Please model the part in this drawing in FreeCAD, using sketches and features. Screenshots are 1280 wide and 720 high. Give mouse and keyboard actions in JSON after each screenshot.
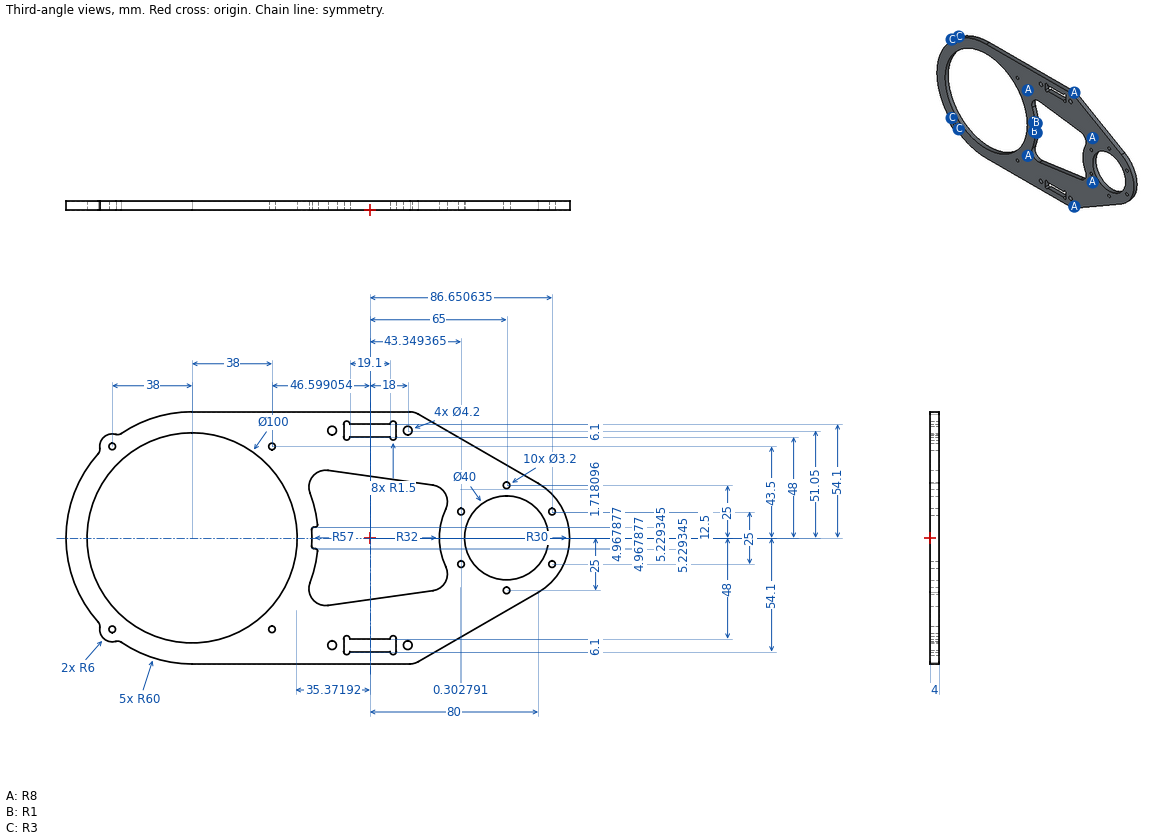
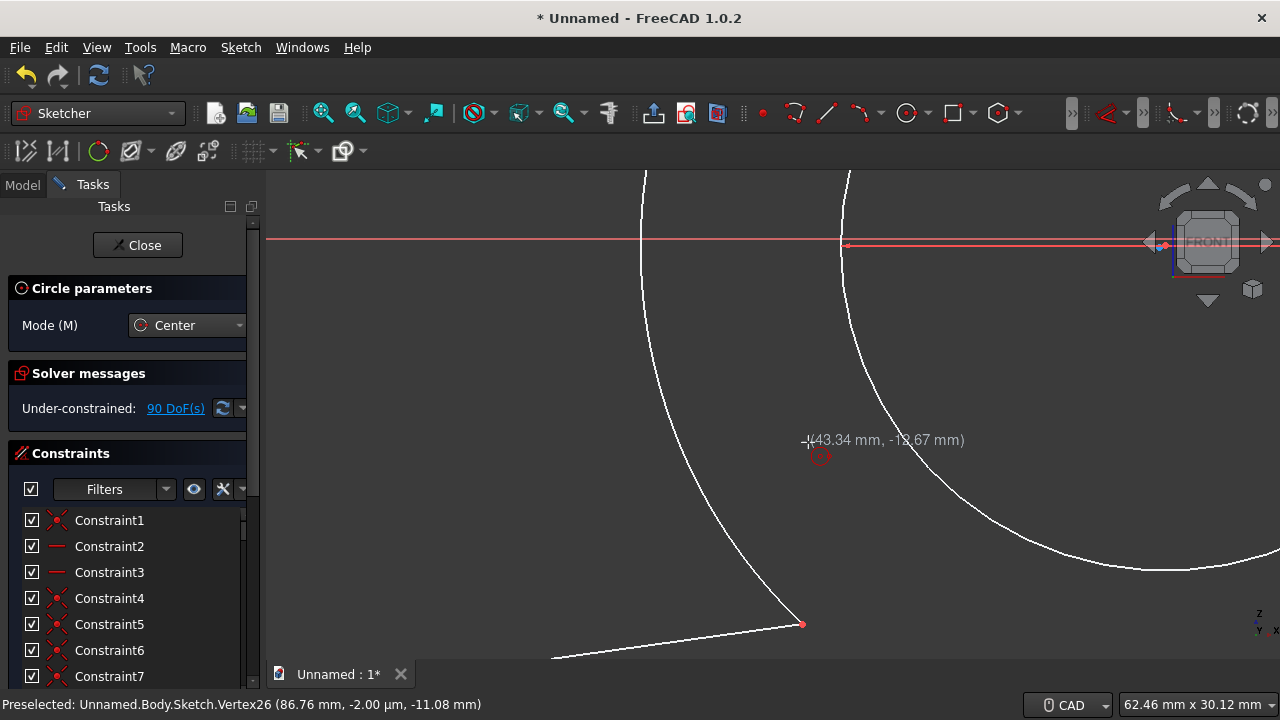
{"action": "scroll", "coordinate": [862, 442], "scroll_direction": "down", "scroll_amount": 10}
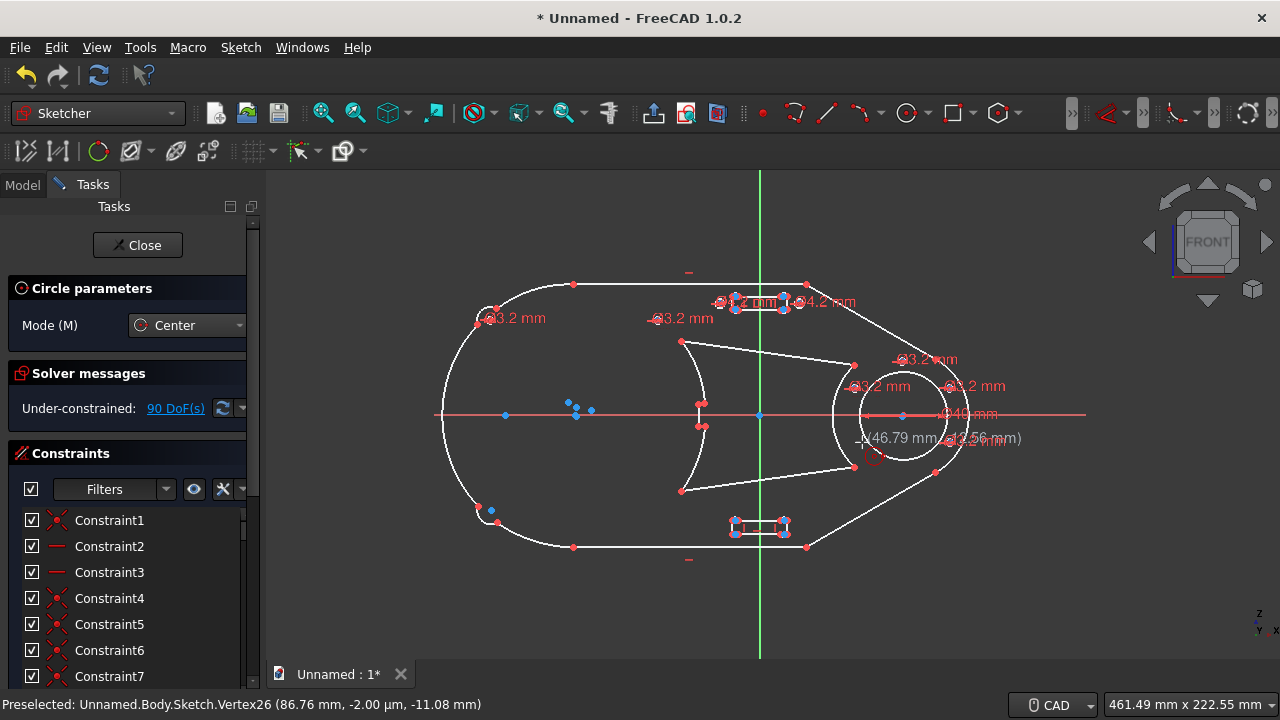
{"action": "scroll", "coordinate": [855, 442], "scroll_direction": "up", "scroll_amount": 2}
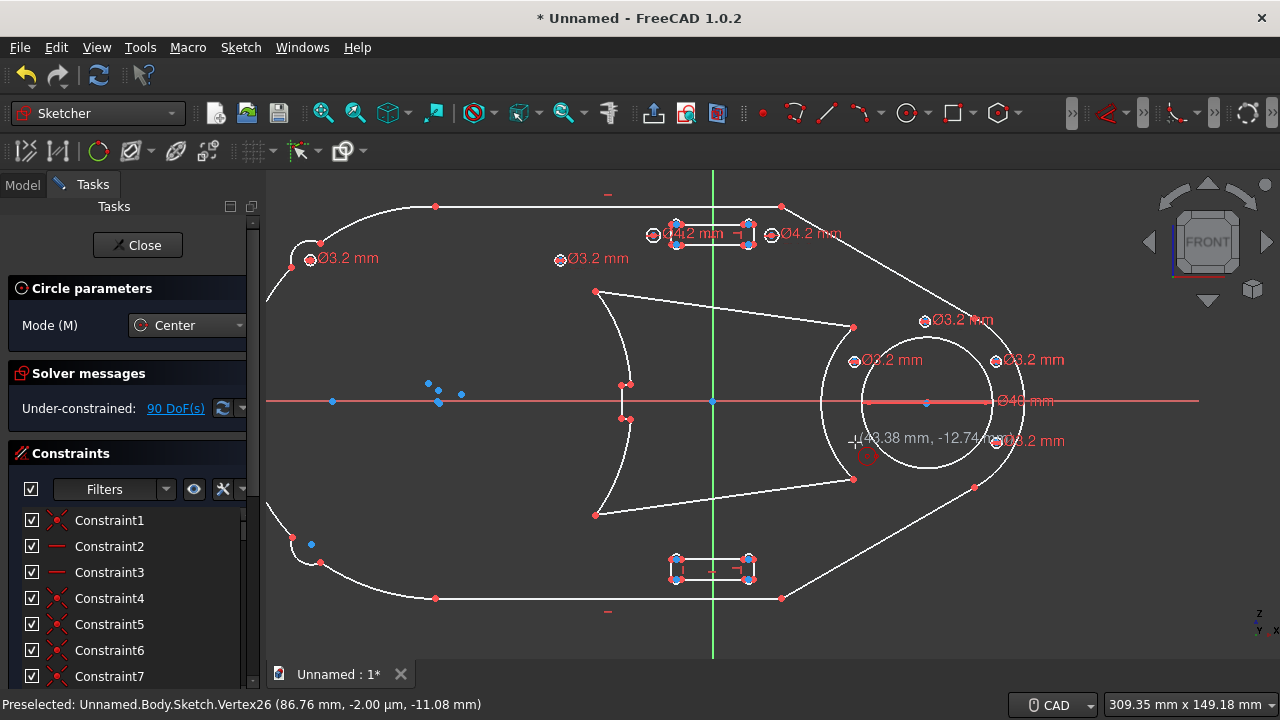
{"action": "left_click", "coordinate": [855, 442]}
{"action": "mouse_move", "coordinate": [851, 439]}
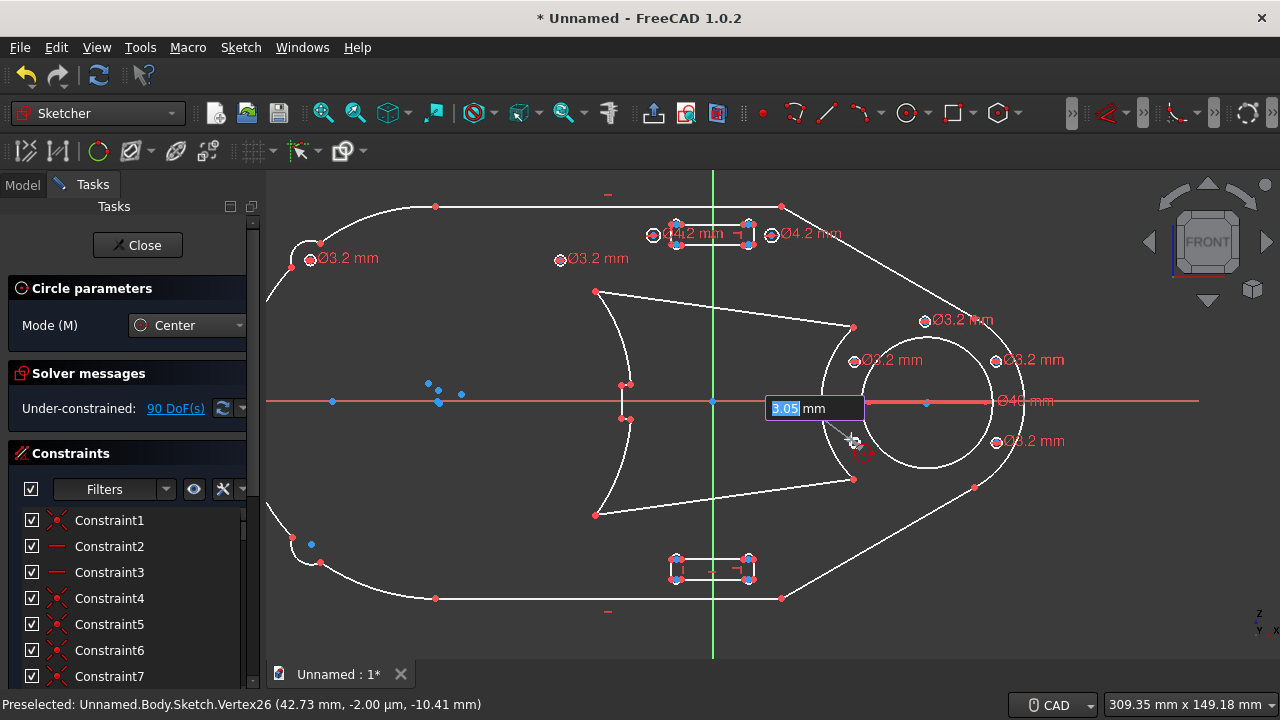
{"action": "type", "text": "3.2"}
{"action": "key", "text": "Return"}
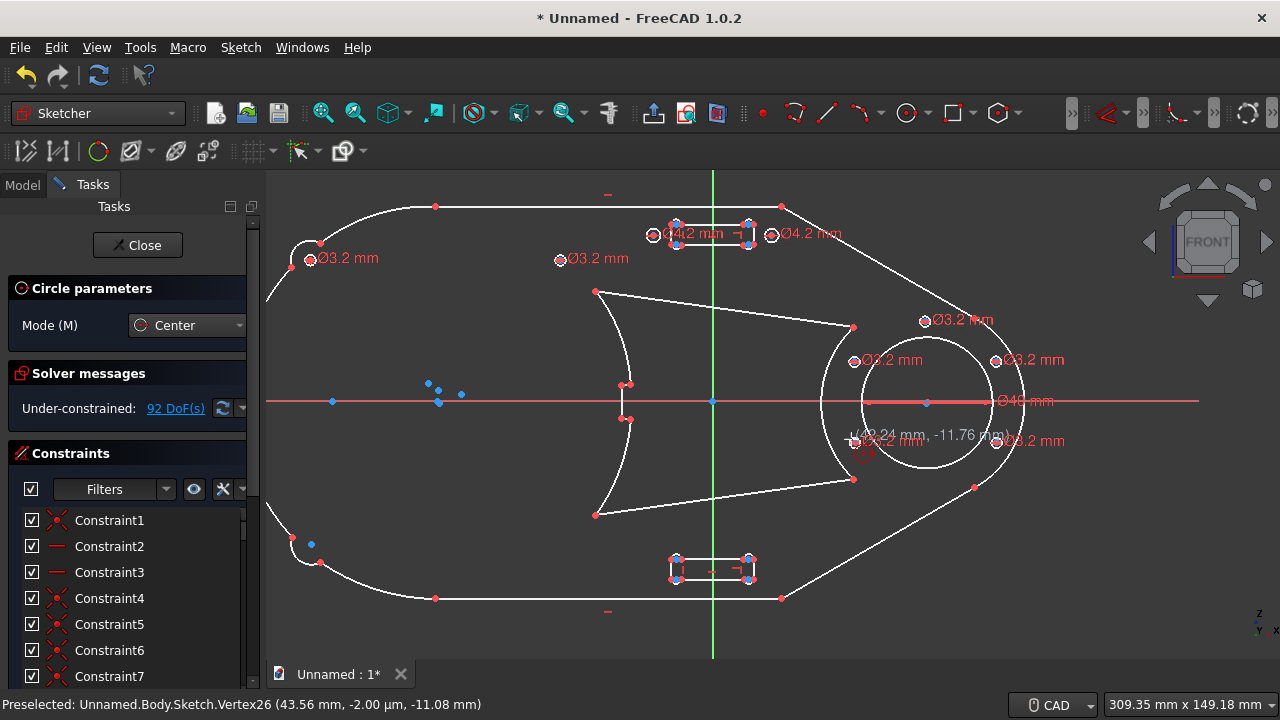
{"action": "scroll", "coordinate": [926, 483], "scroll_direction": "up", "scroll_amount": 8}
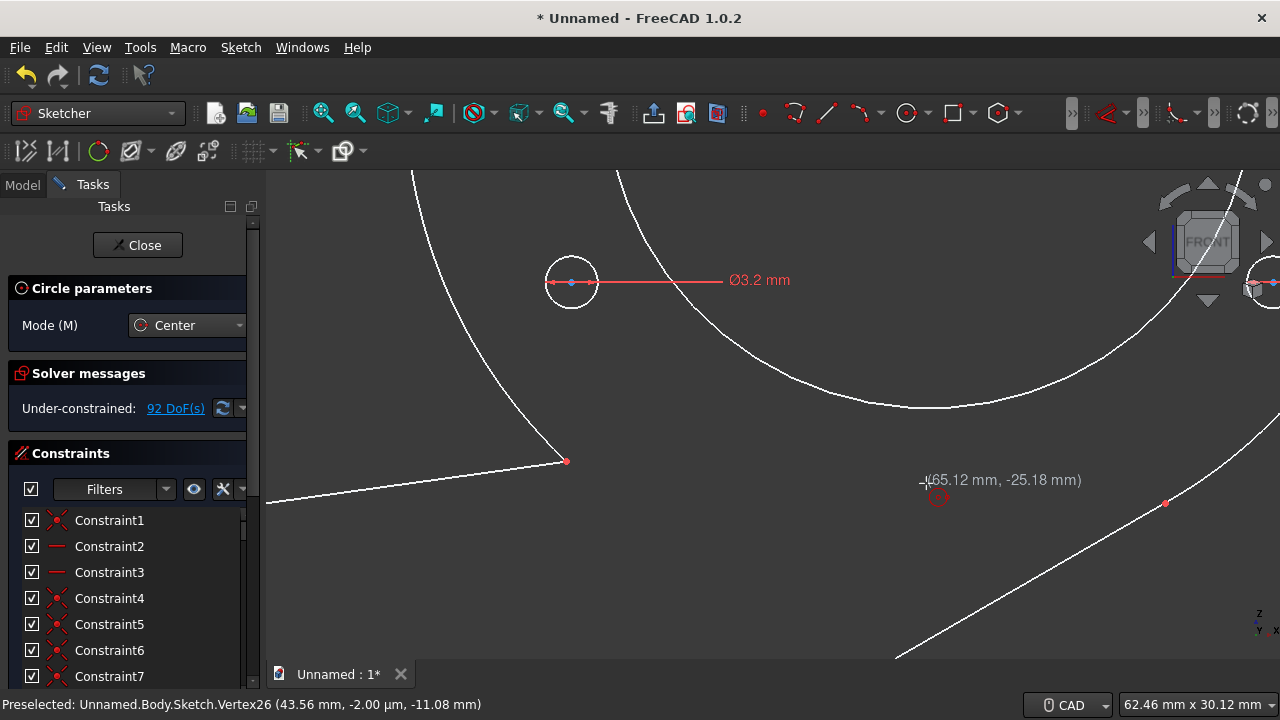
{"action": "scroll", "coordinate": [899, 467], "scroll_direction": "down", "scroll_amount": 10}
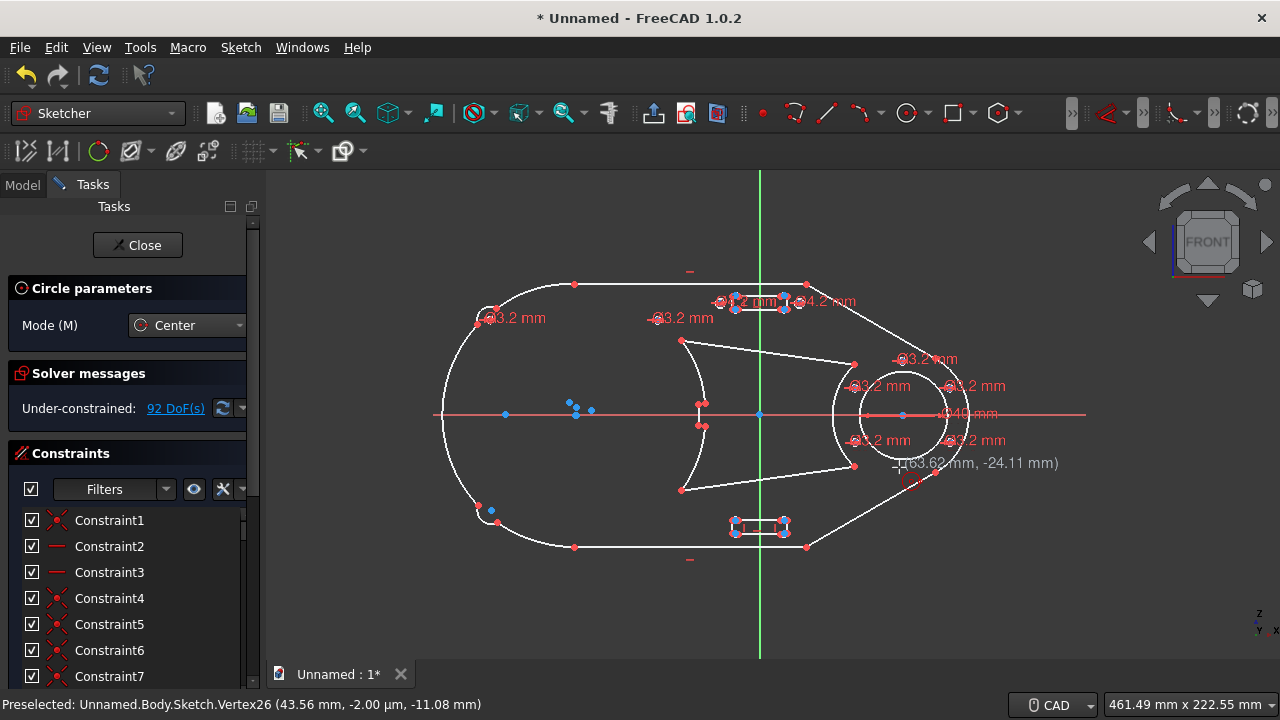
{"action": "scroll", "coordinate": [903, 470], "scroll_direction": "up", "scroll_amount": 2}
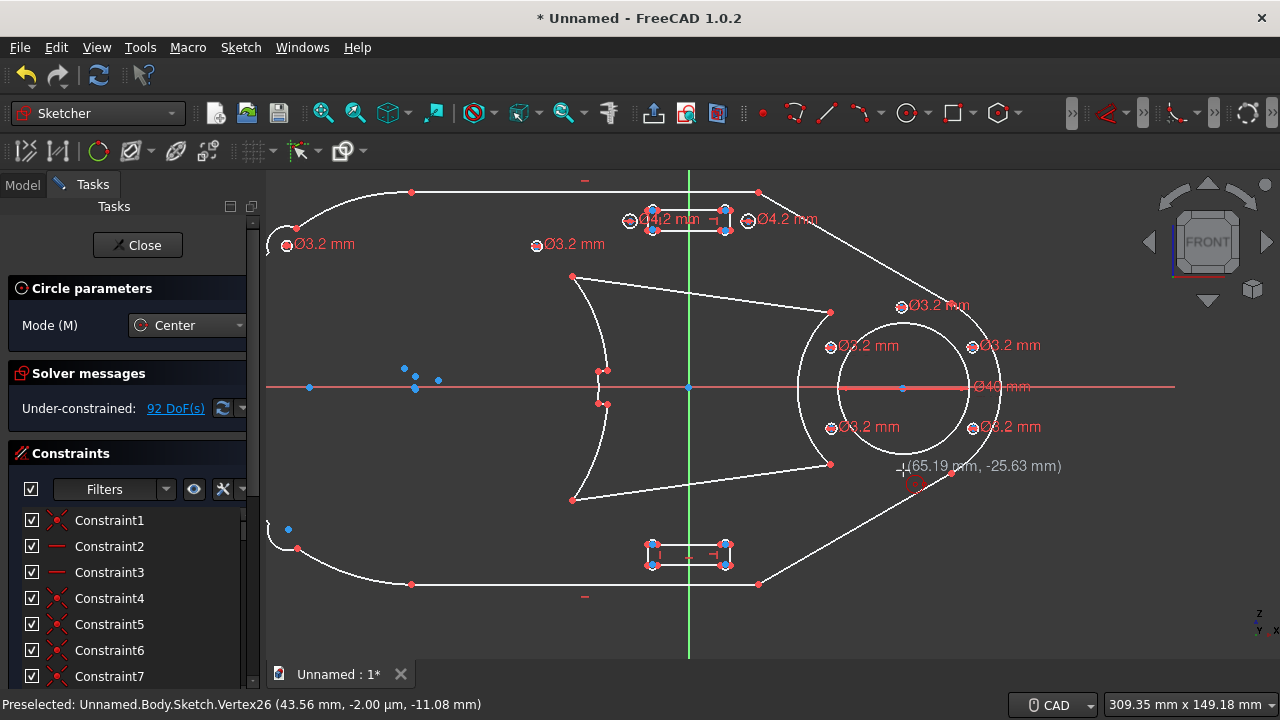
{"action": "left_click", "coordinate": [902, 469]}
{"action": "mouse_move", "coordinate": [906, 473]}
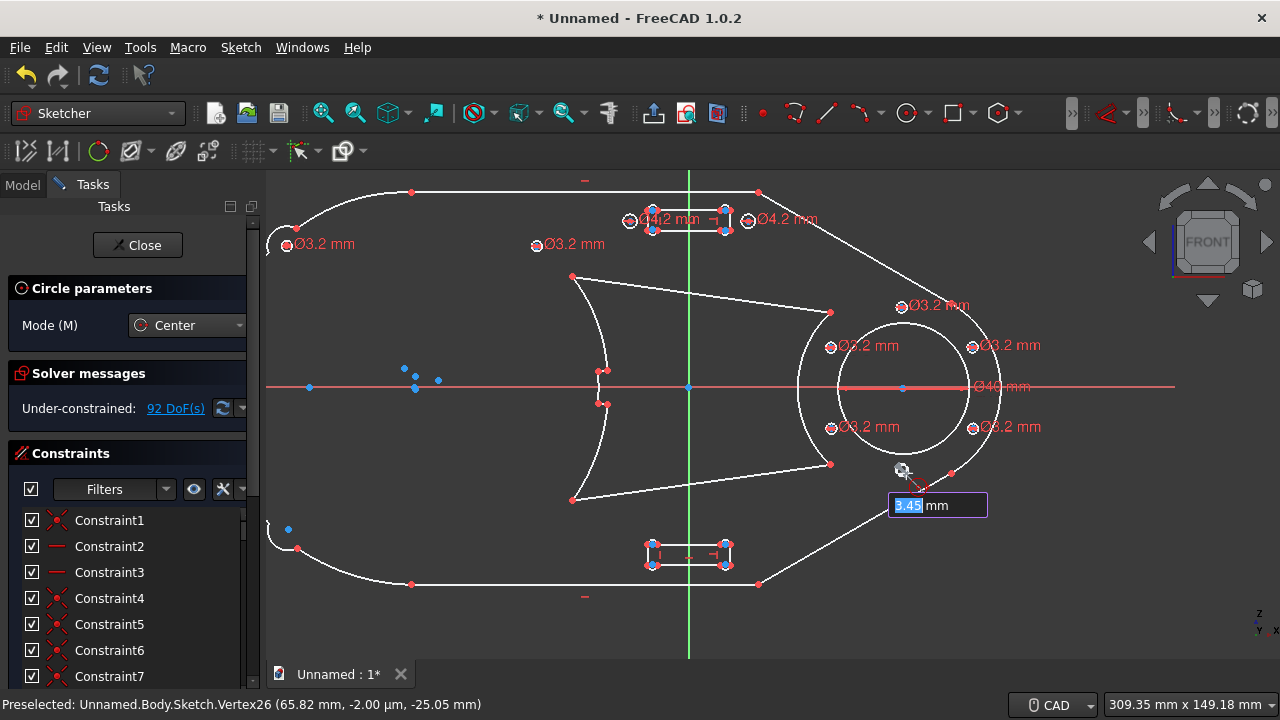
{"action": "type", "text": "3.2"}
{"action": "key", "text": "Return"}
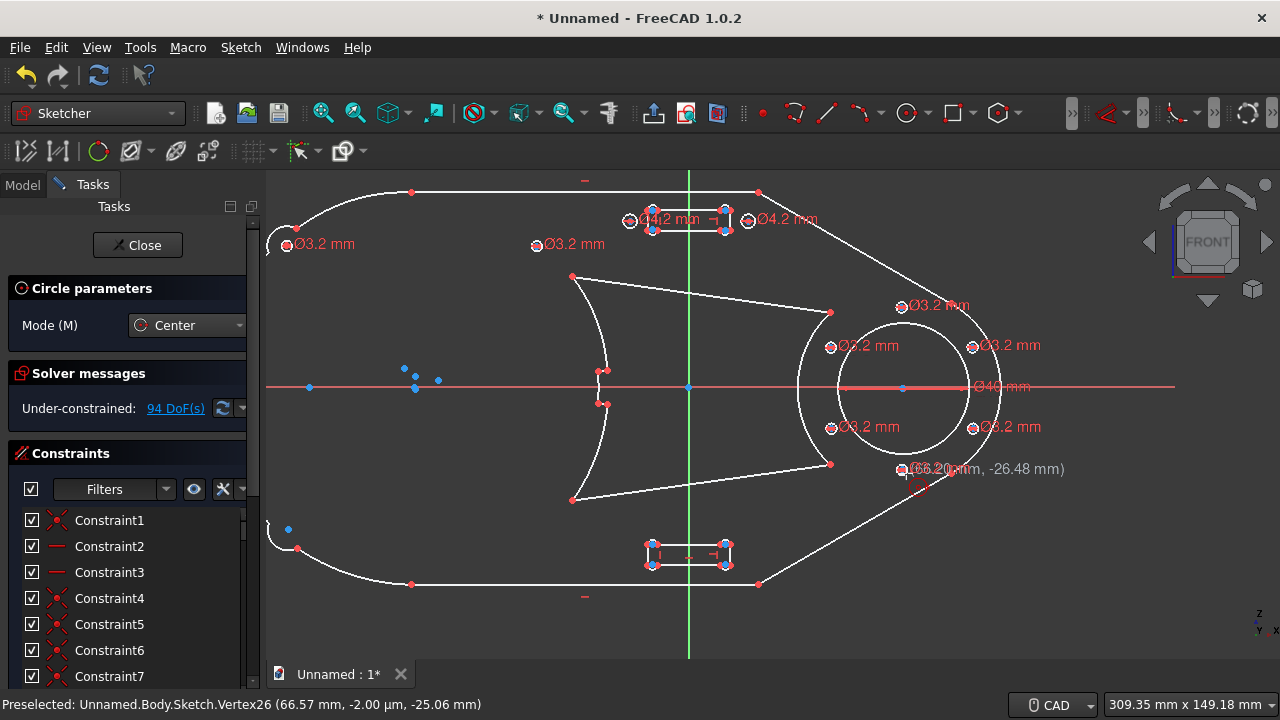
{"action": "scroll", "coordinate": [748, 555], "scroll_direction": "up", "scroll_amount": 6}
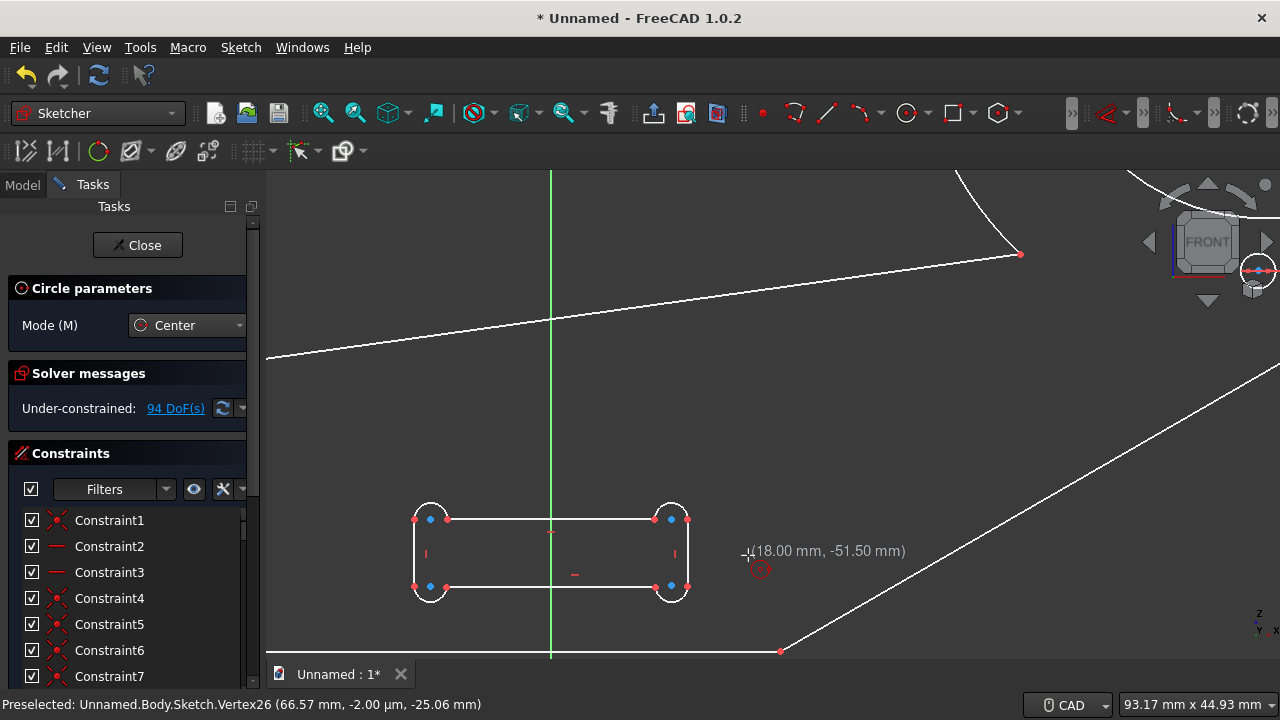
{"action": "scroll", "coordinate": [812, 520], "scroll_direction": "down", "scroll_amount": 8}